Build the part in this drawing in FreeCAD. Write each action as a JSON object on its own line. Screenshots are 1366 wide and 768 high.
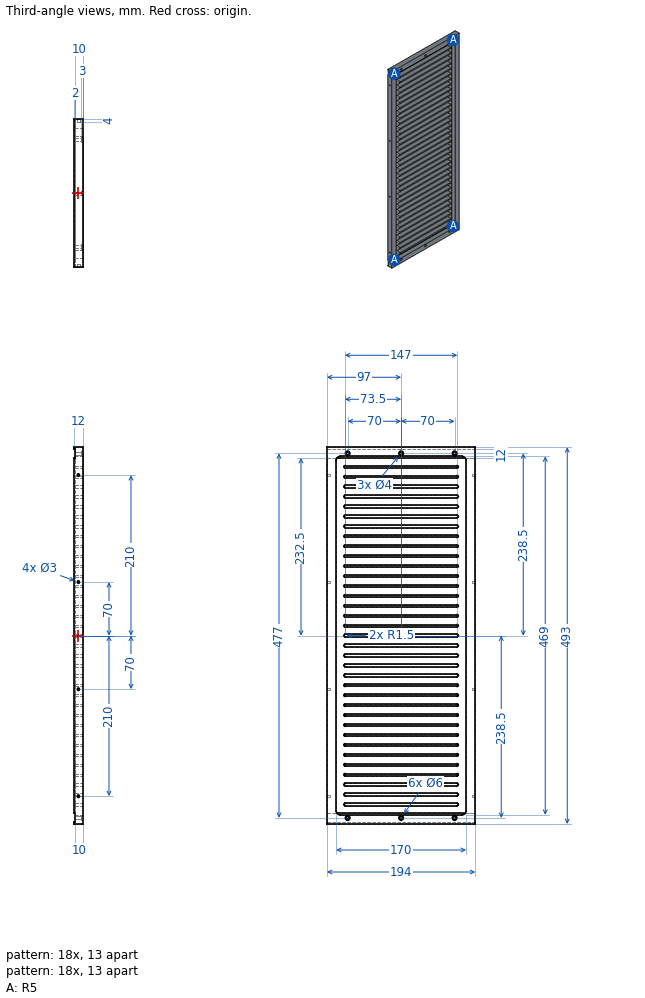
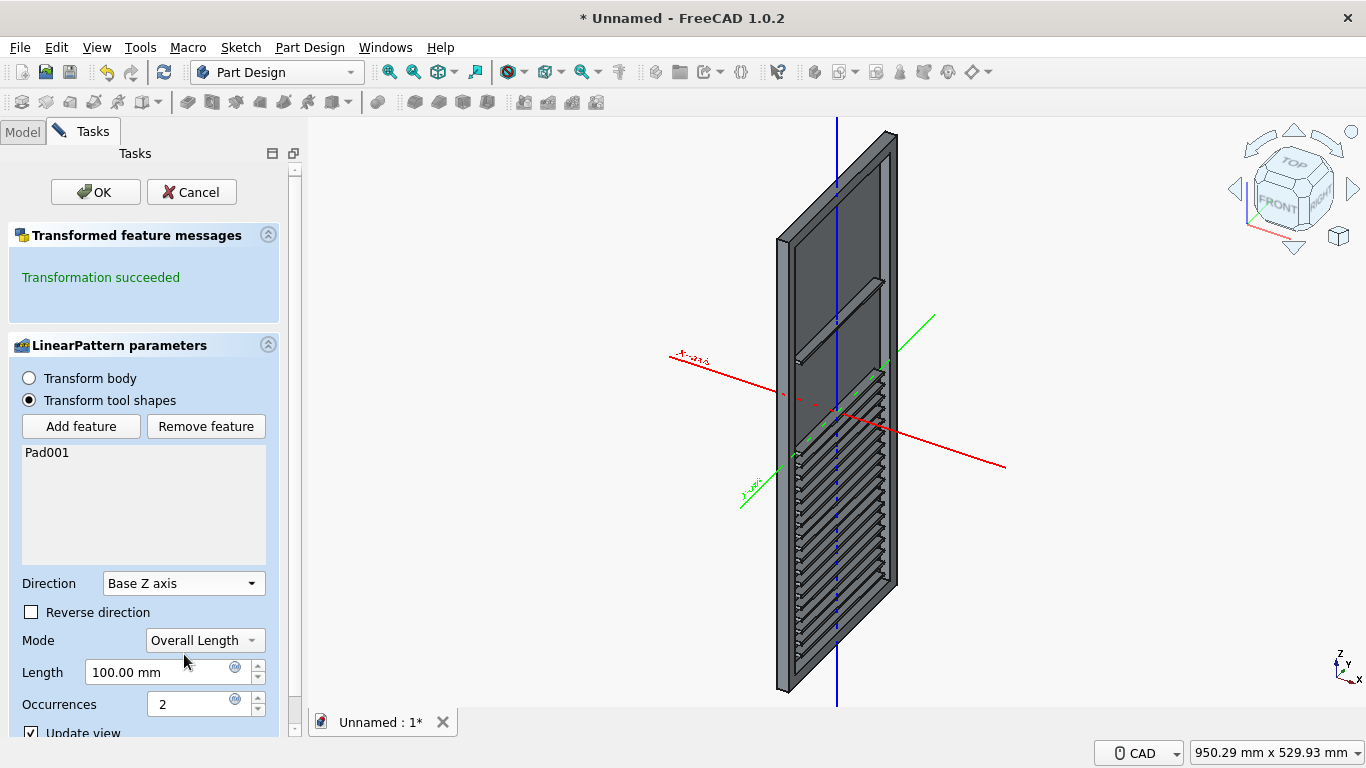
{"action": "left_click", "coordinate": [206, 640]}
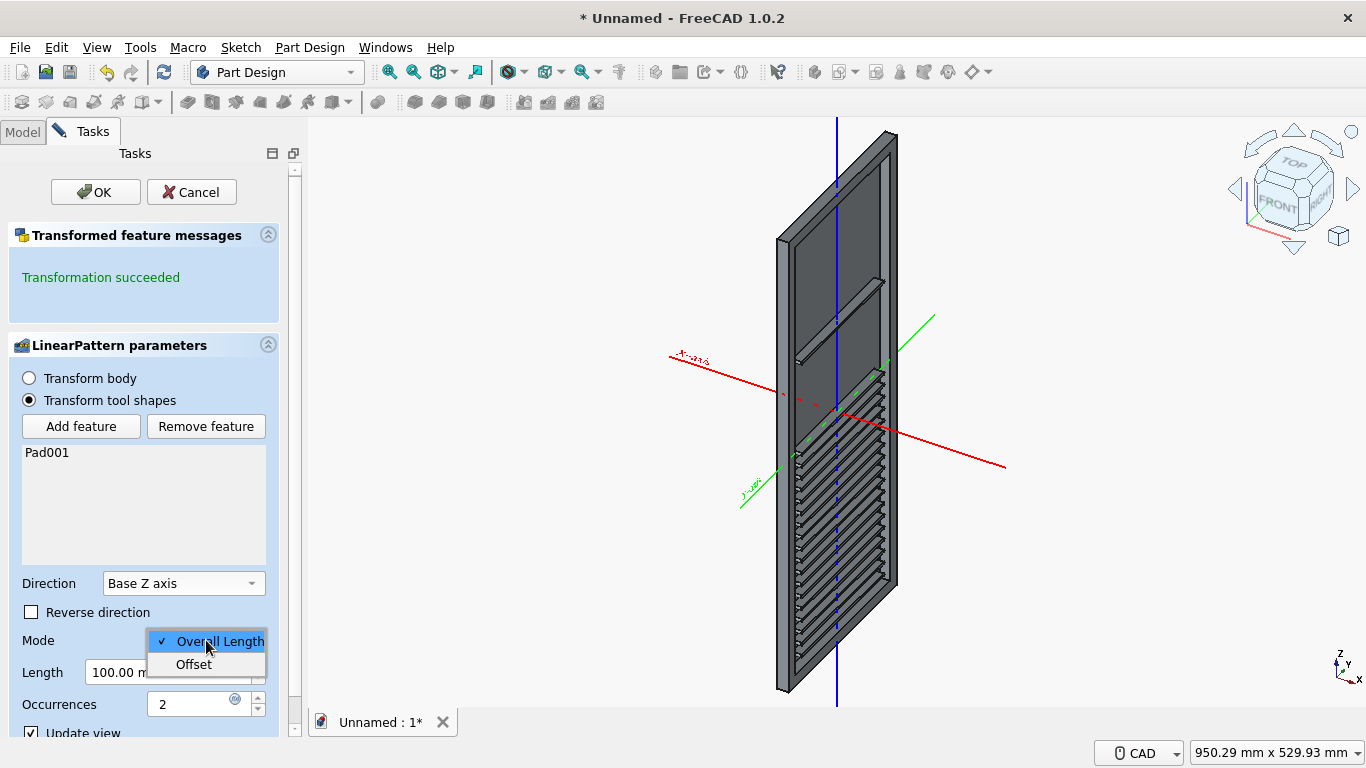
{"action": "left_click", "coordinate": [206, 664]}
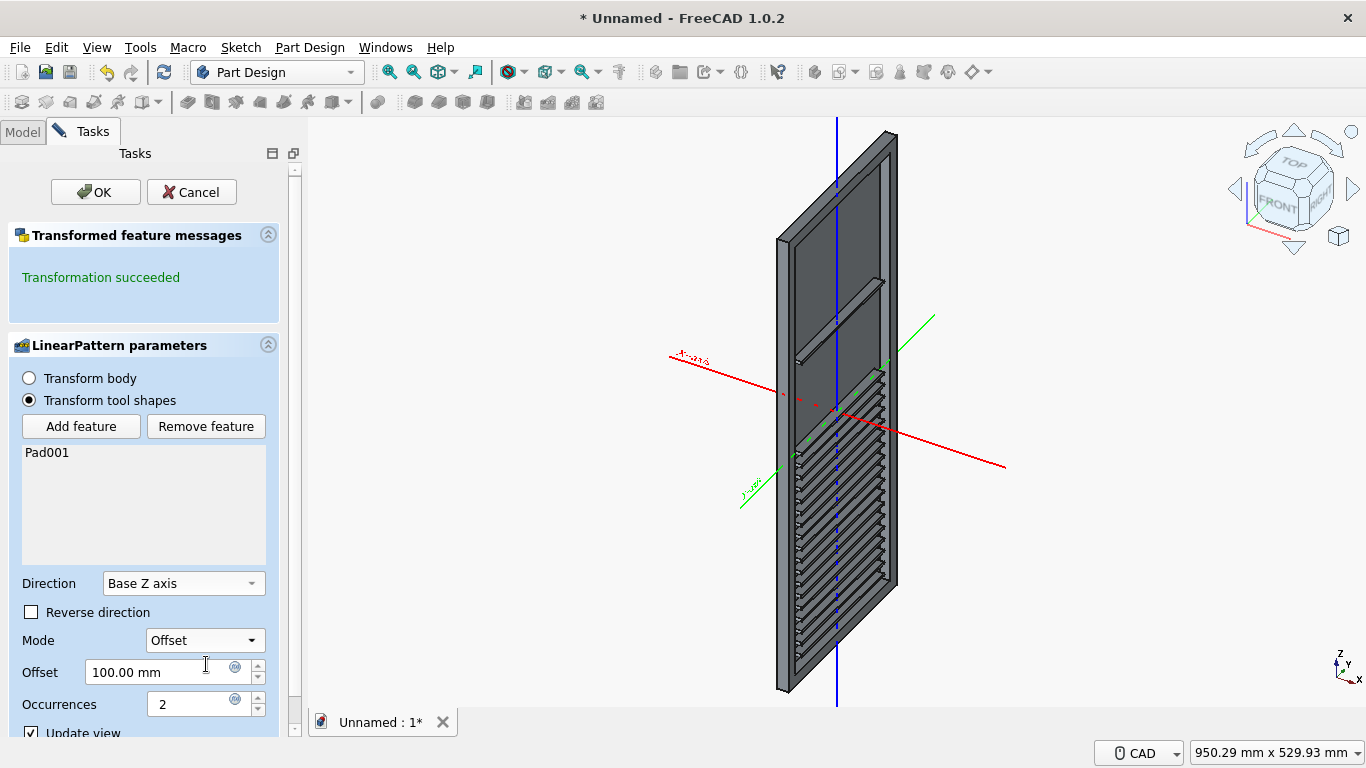
{"action": "triple_click", "coordinate": [168, 672]}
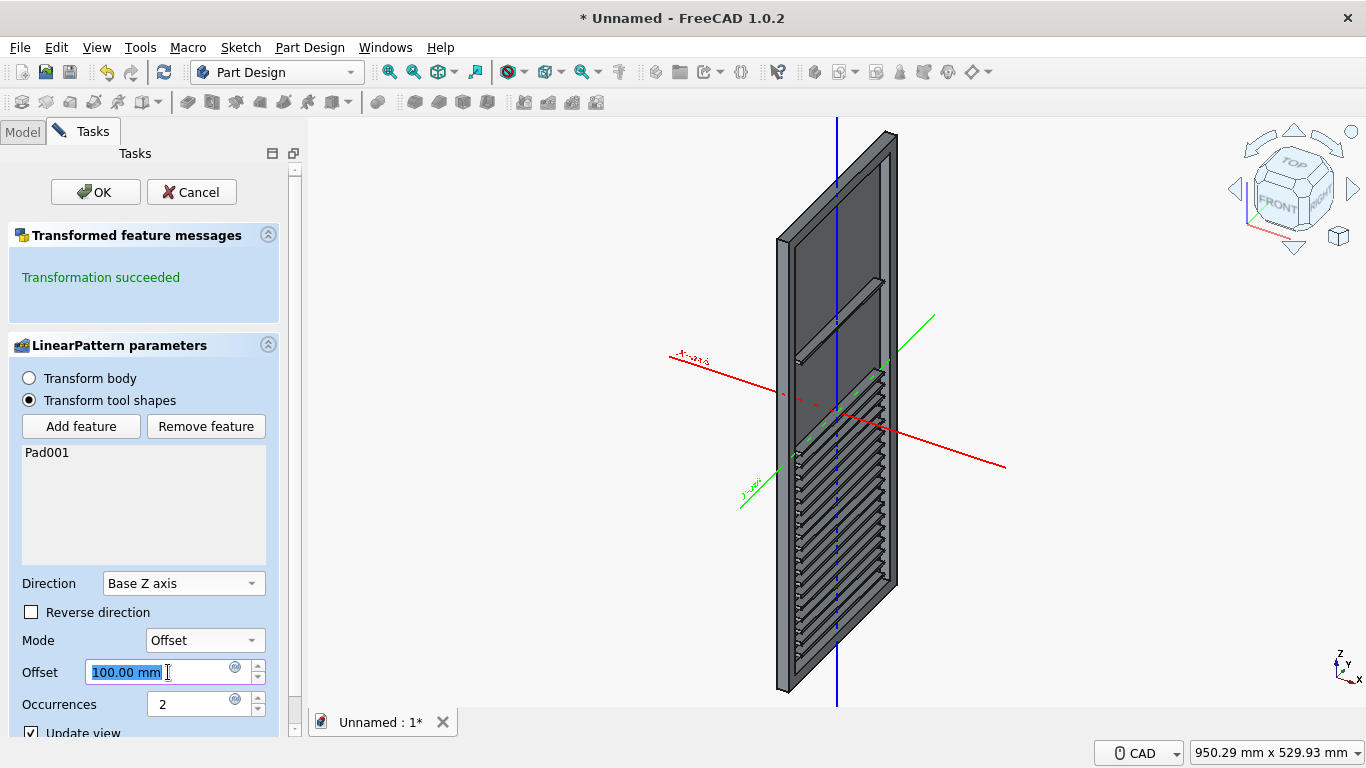
{"action": "type", "text": "13"}
{"action": "key", "text": "Tab"}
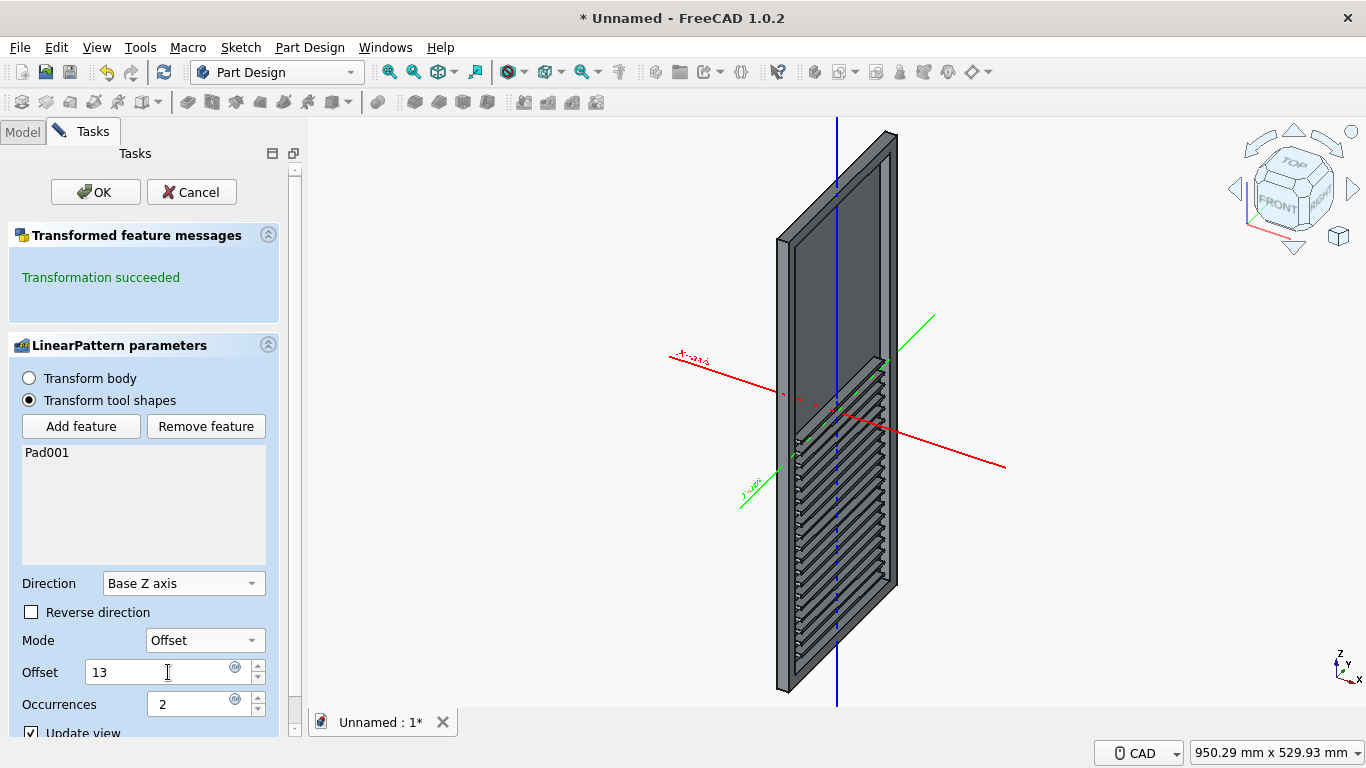
{"action": "triple_click", "coordinate": [198, 704]}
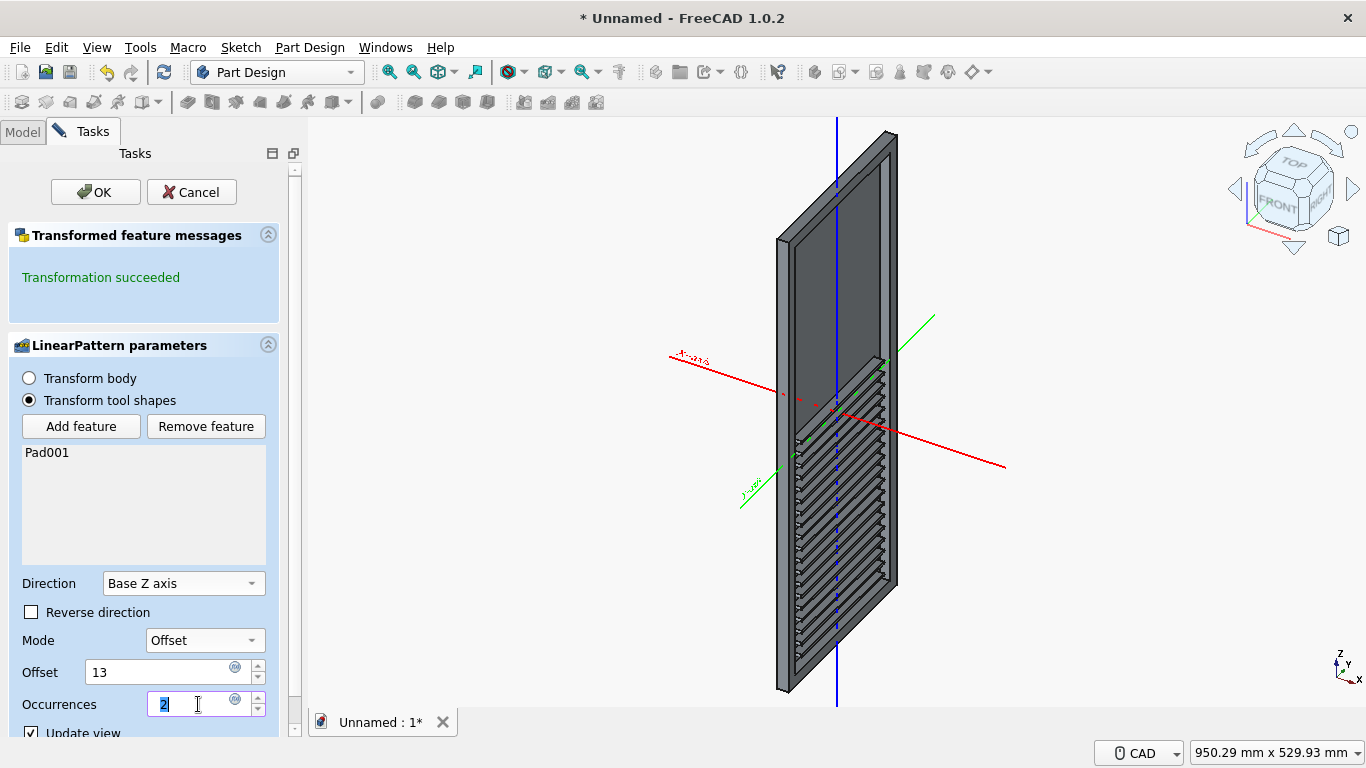
{"action": "type", "text": "18"}
{"action": "key", "text": "Tab"}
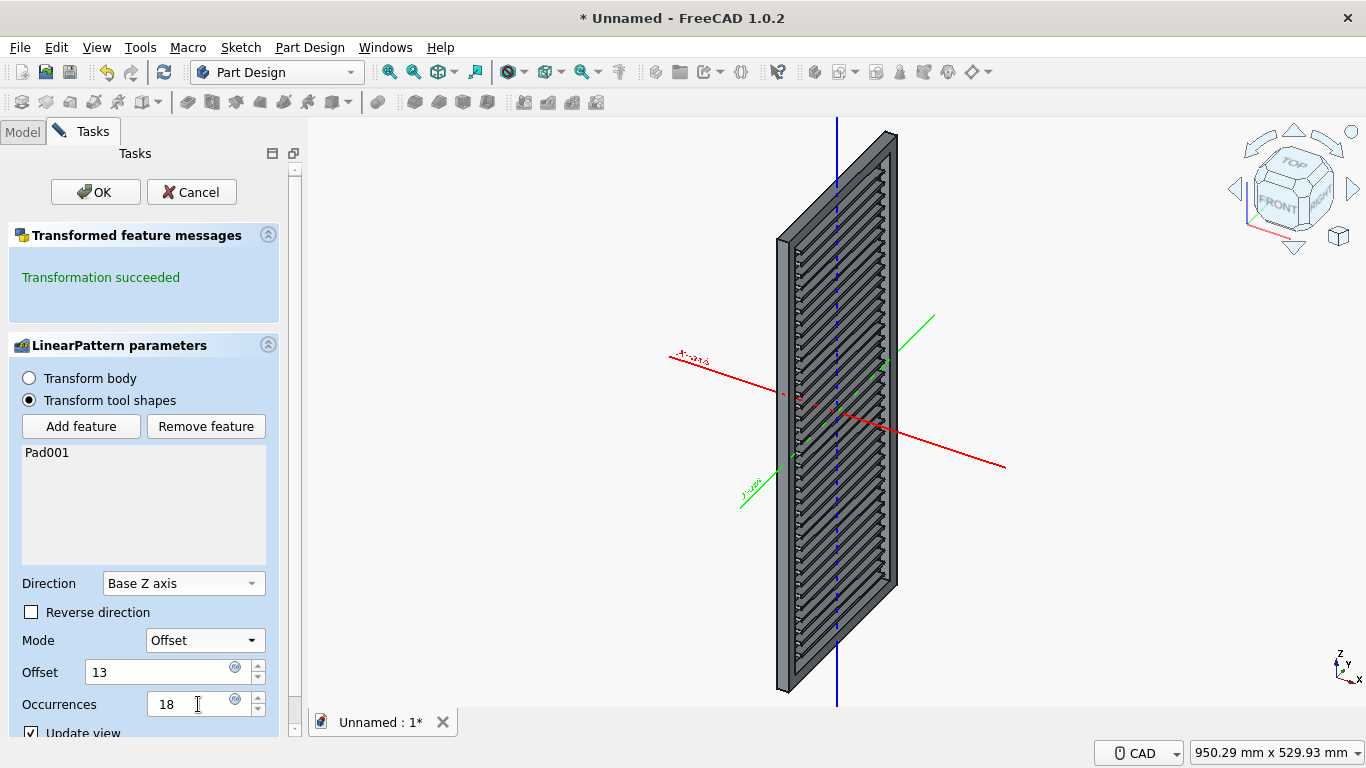
{"action": "left_click", "coordinate": [96, 192]}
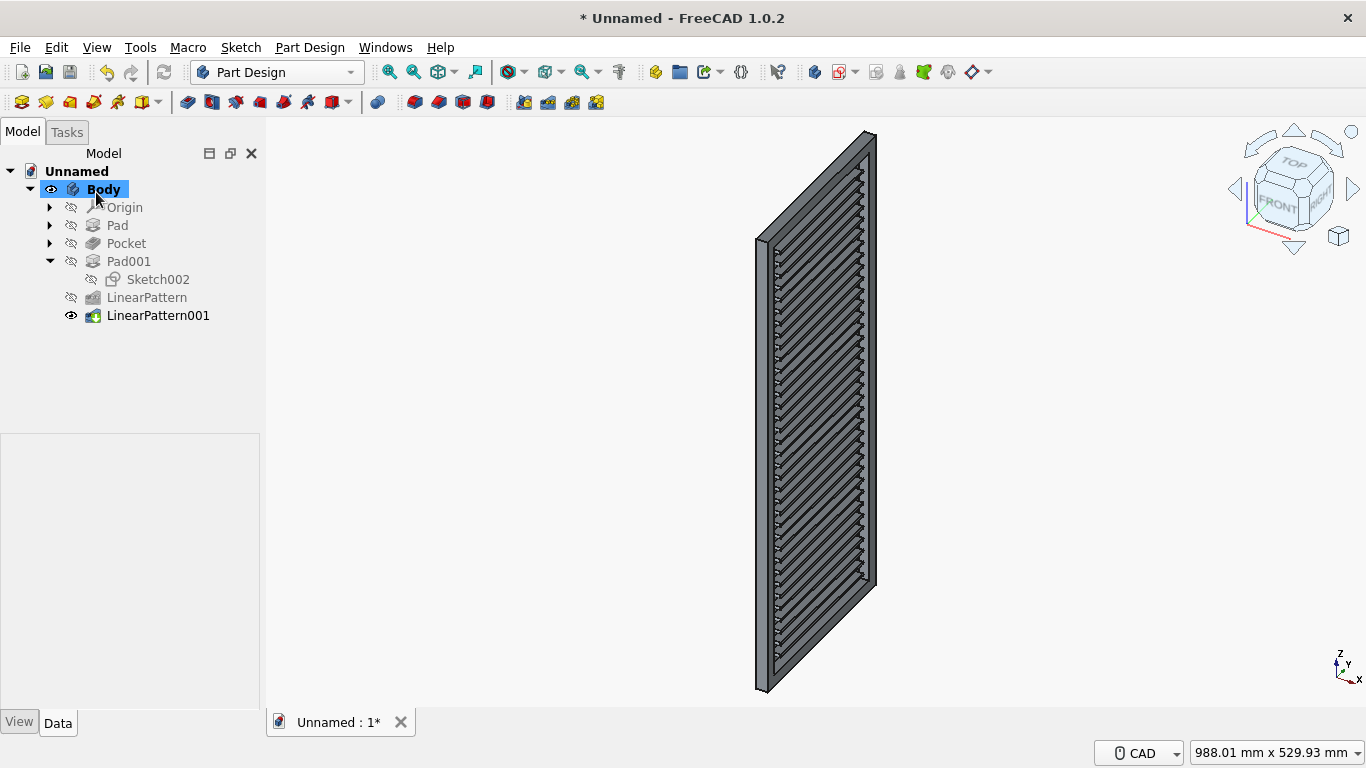
{"action": "scroll", "coordinate": [770, 672], "scroll_direction": "up", "scroll_amount": 7}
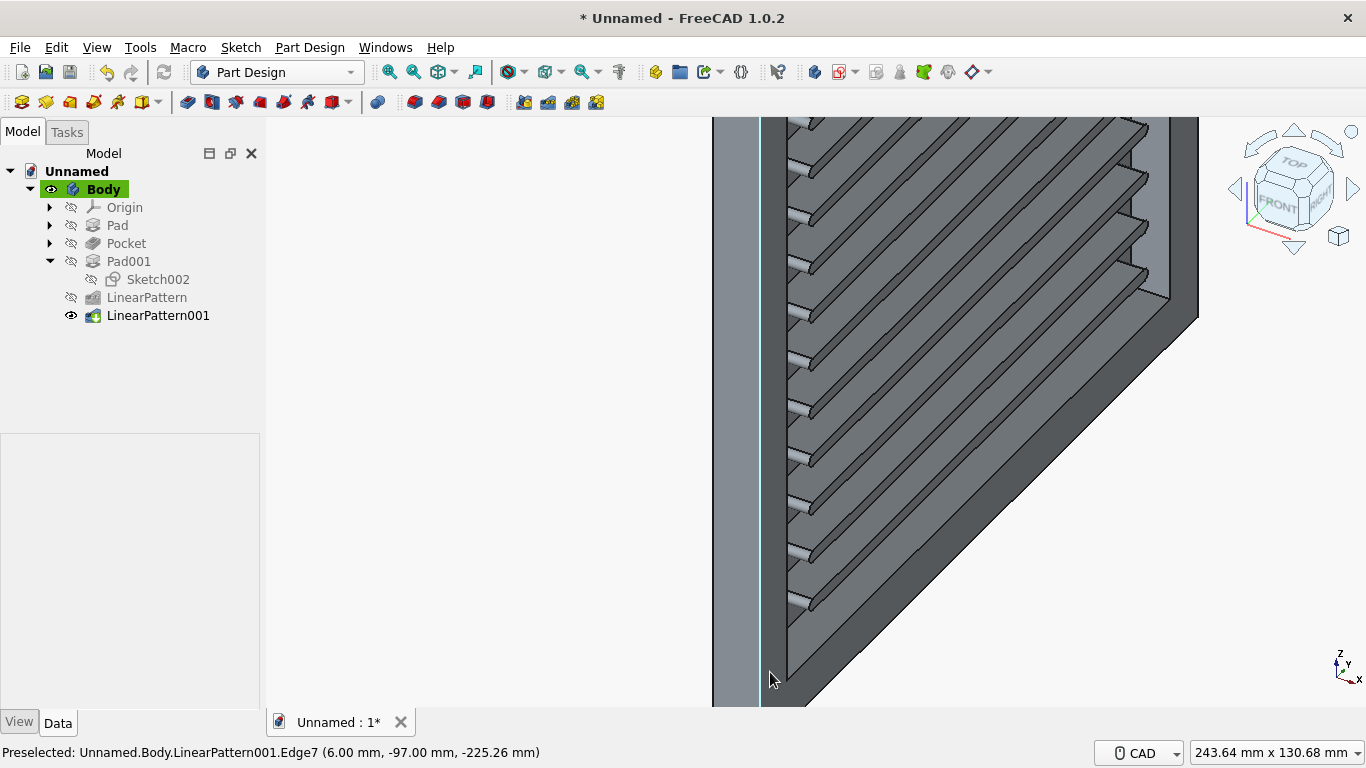
{"action": "left_click", "coordinate": [390, 72]}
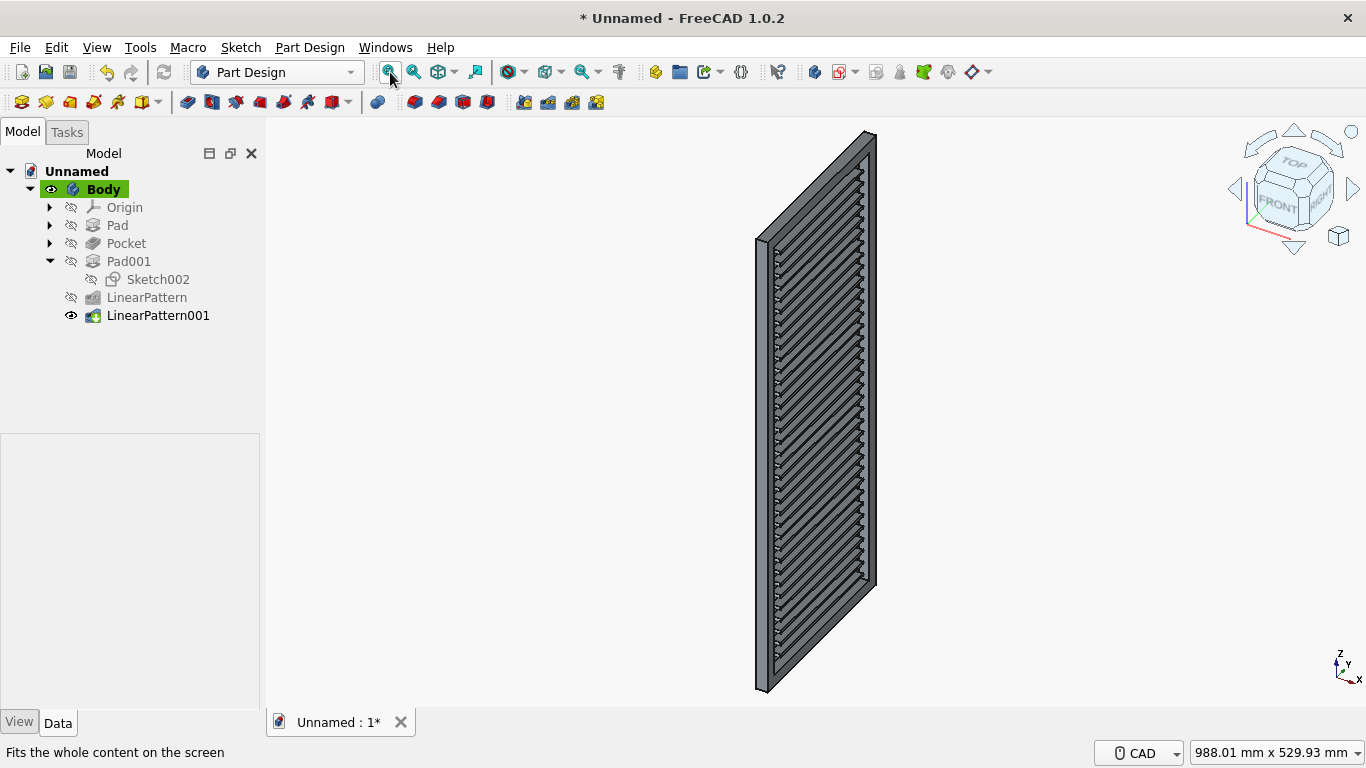
{"action": "key", "text": "0"}